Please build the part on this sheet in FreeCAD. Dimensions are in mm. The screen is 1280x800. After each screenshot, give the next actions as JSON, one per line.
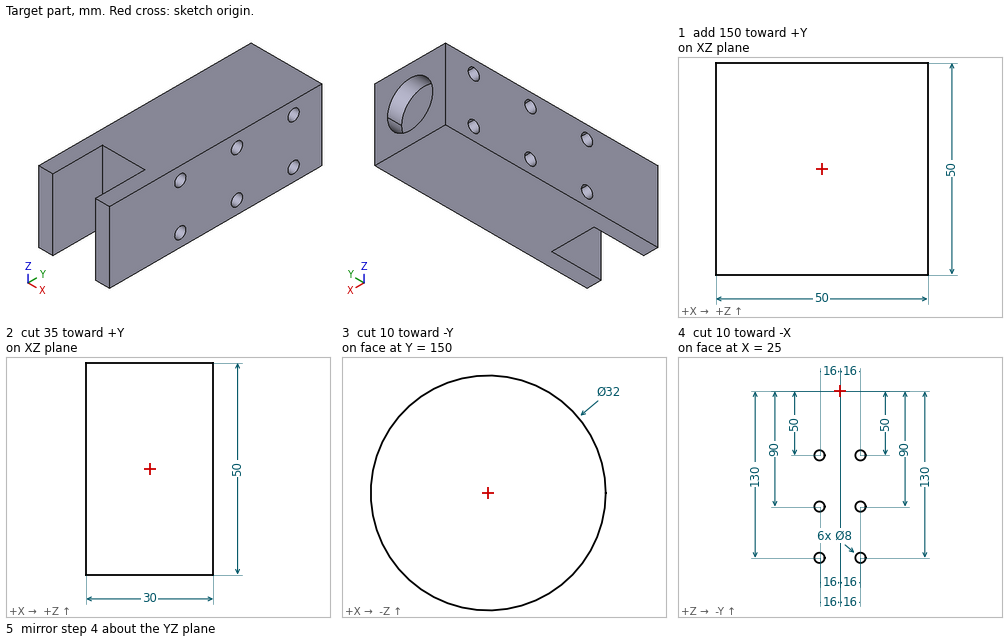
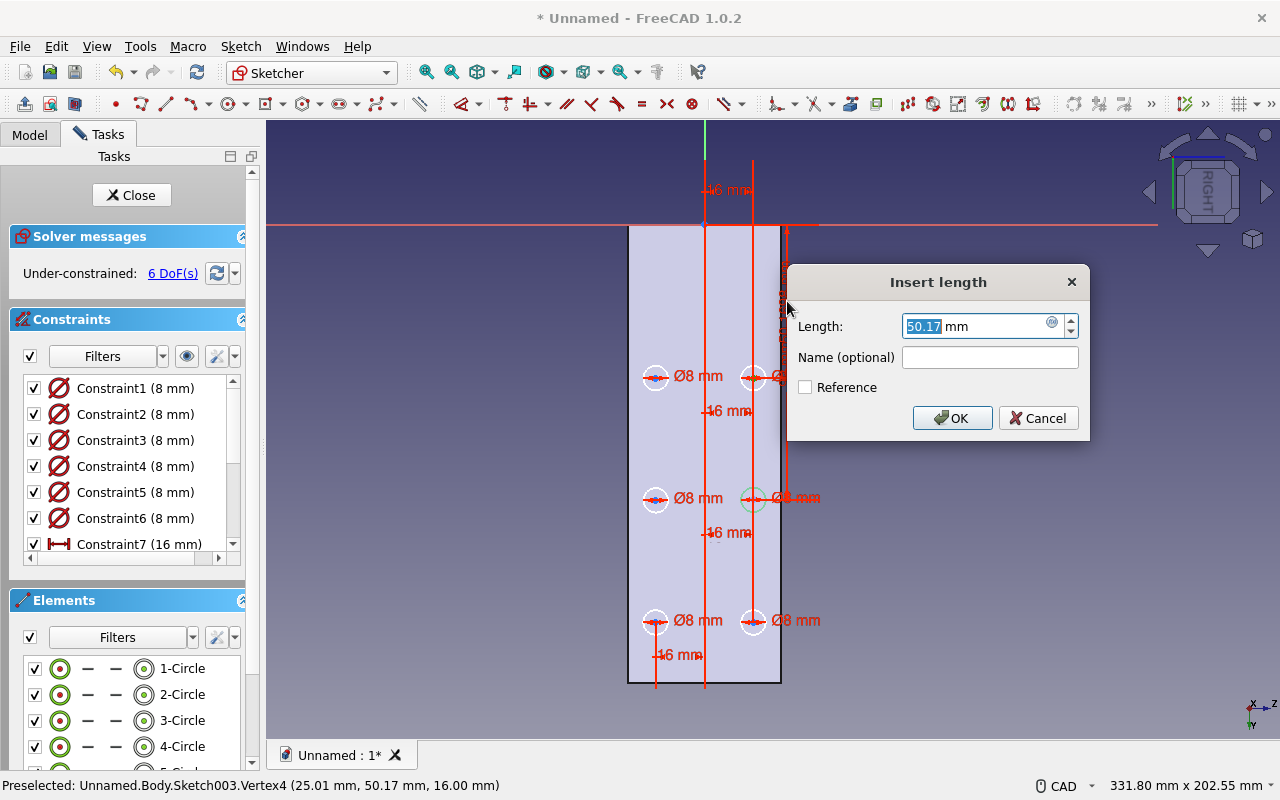
{"action": "type", "text": "50"}
{"action": "key", "text": "Return"}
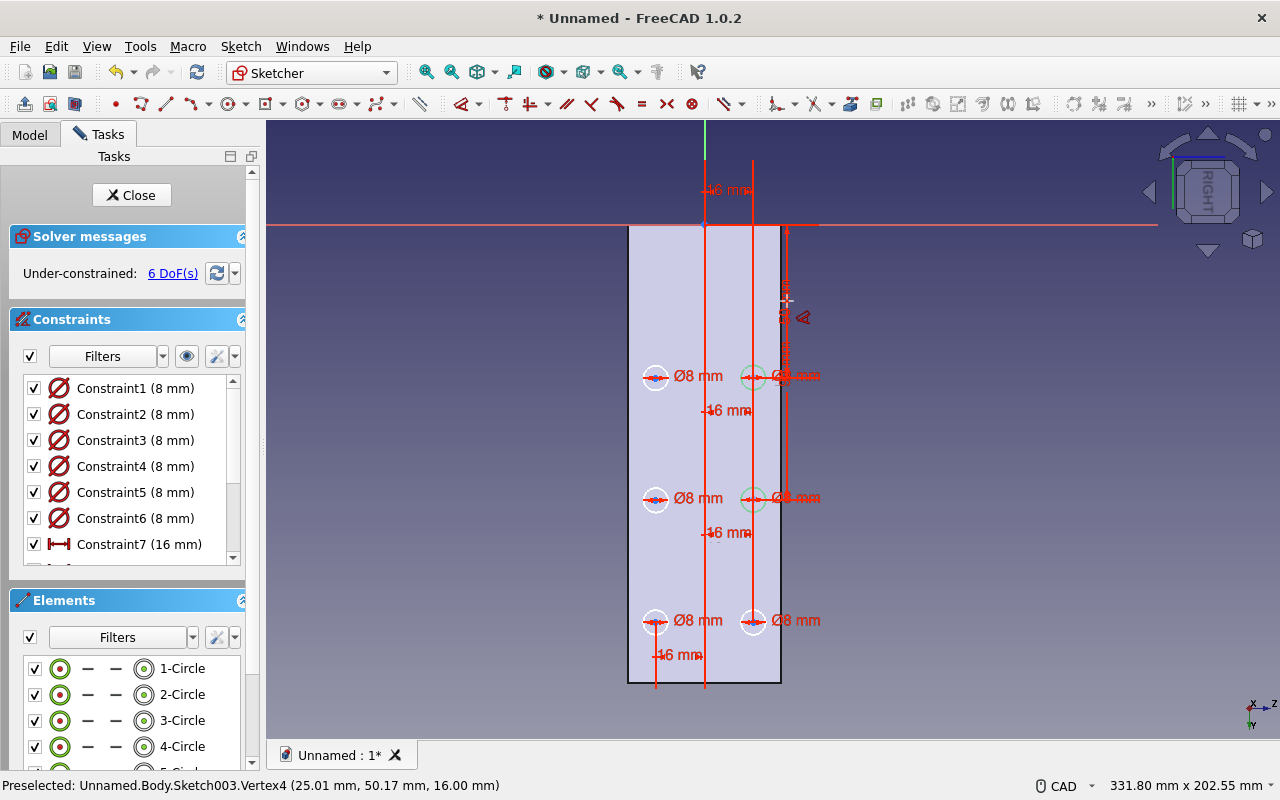
{"action": "left_click", "coordinate": [656, 378]}
{"action": "left_click", "coordinate": [680, 167]}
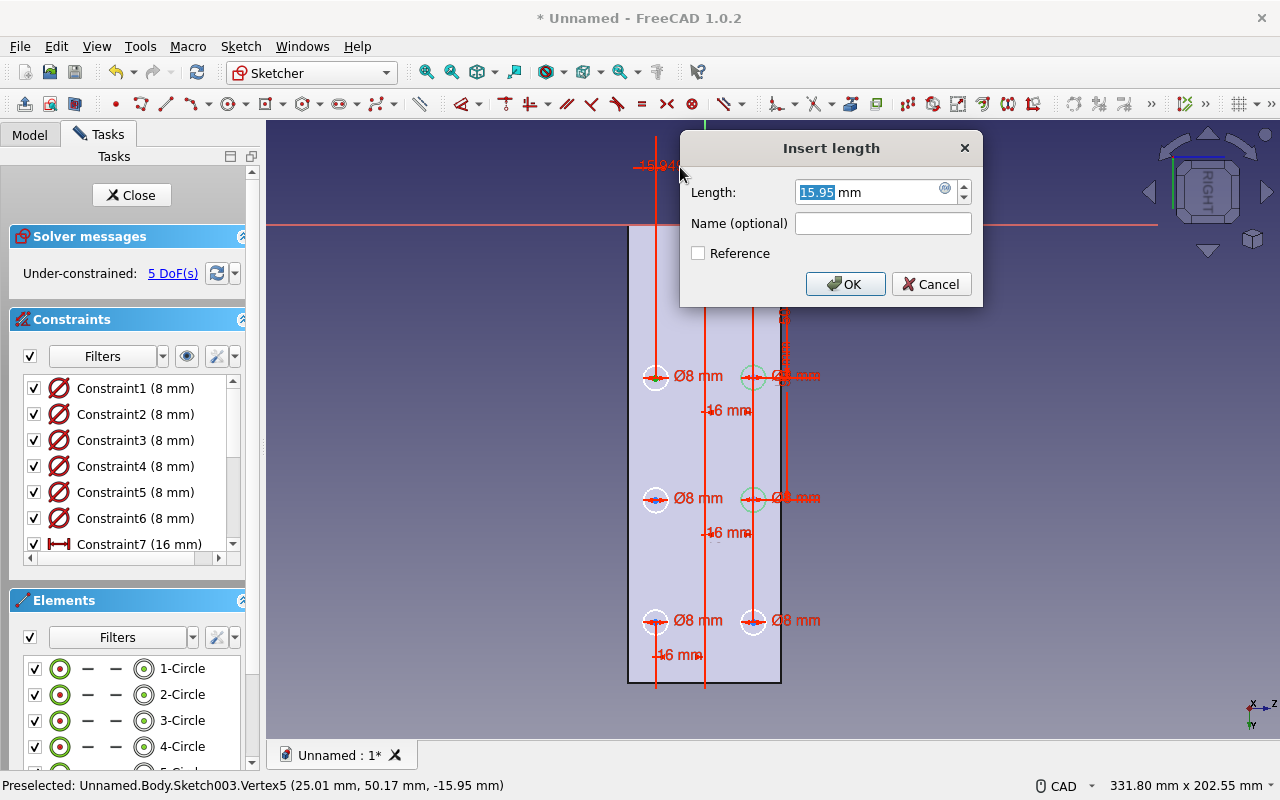
{"action": "type", "text": "16"}
{"action": "key", "text": "Return"}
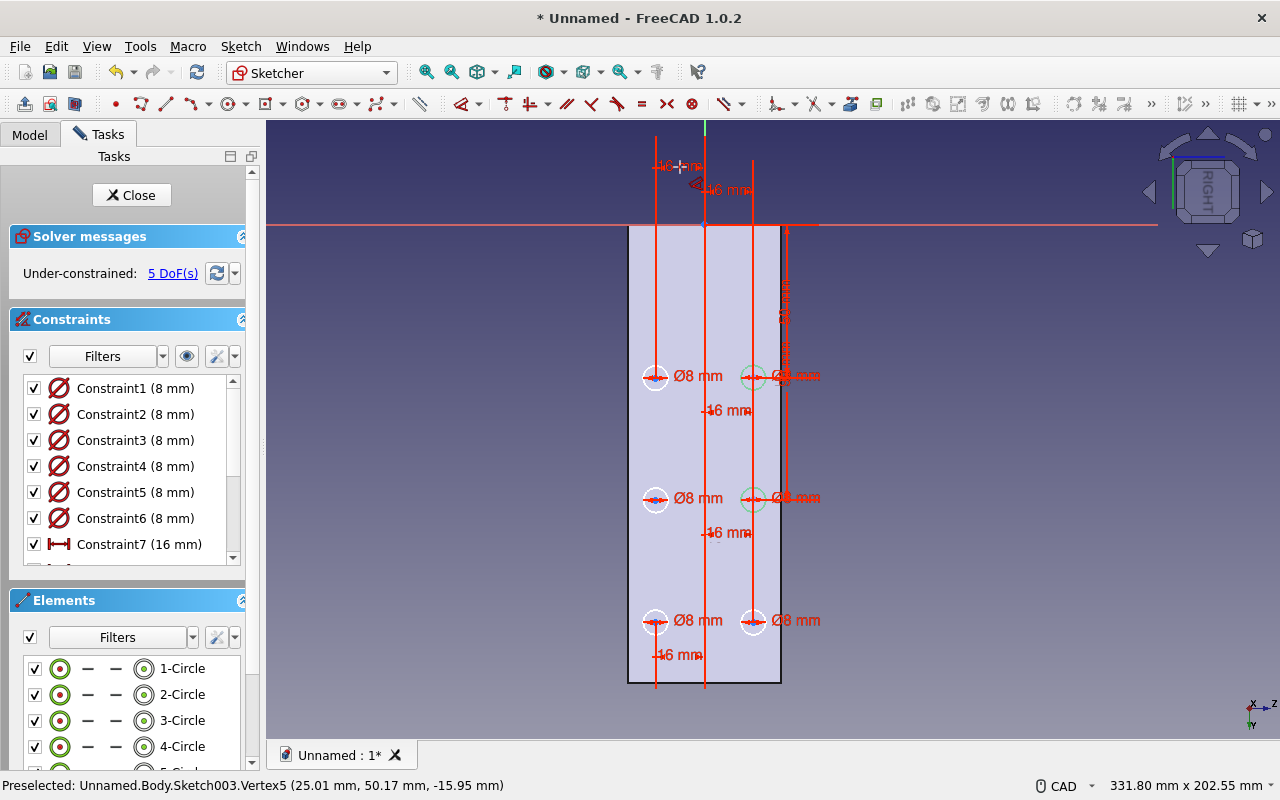
{"action": "left_click", "coordinate": [656, 378]}
{"action": "left_click", "coordinate": [622, 301]}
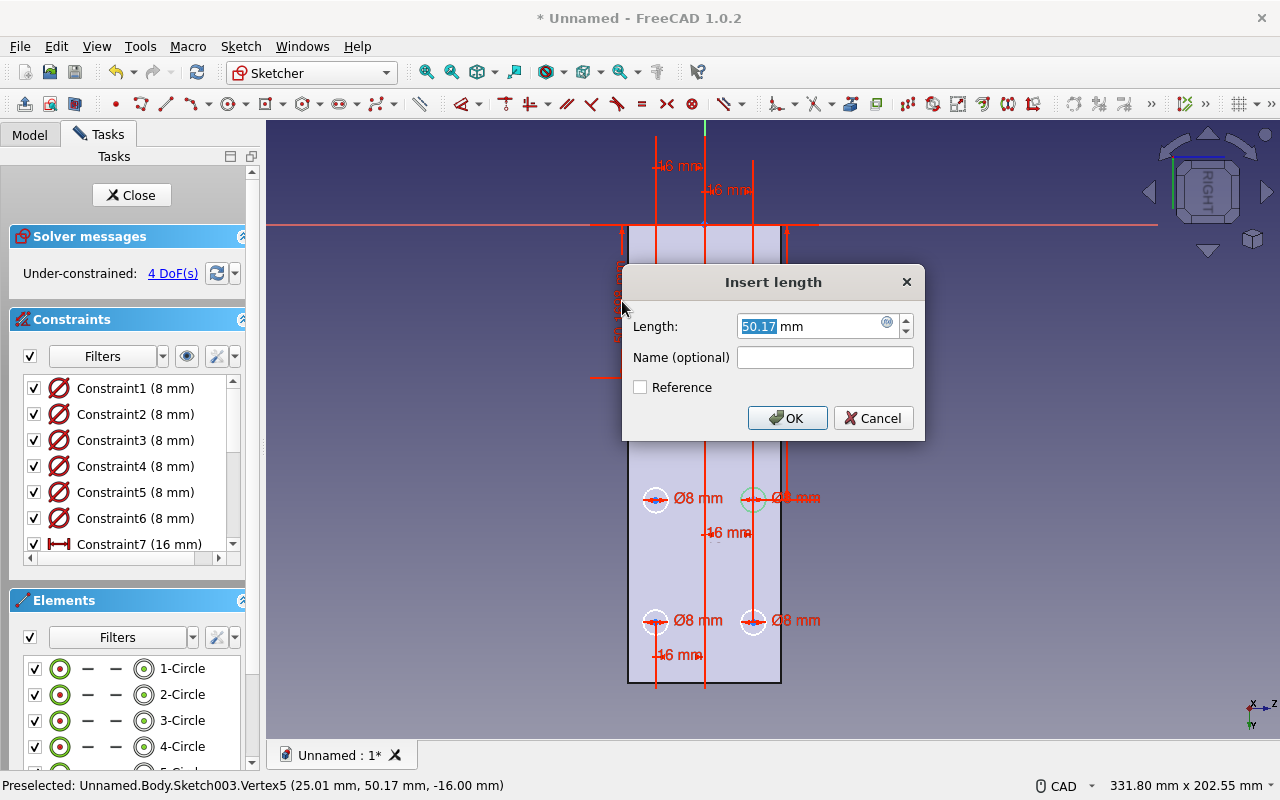
{"action": "type", "text": "50"}
{"action": "key", "text": "Return"}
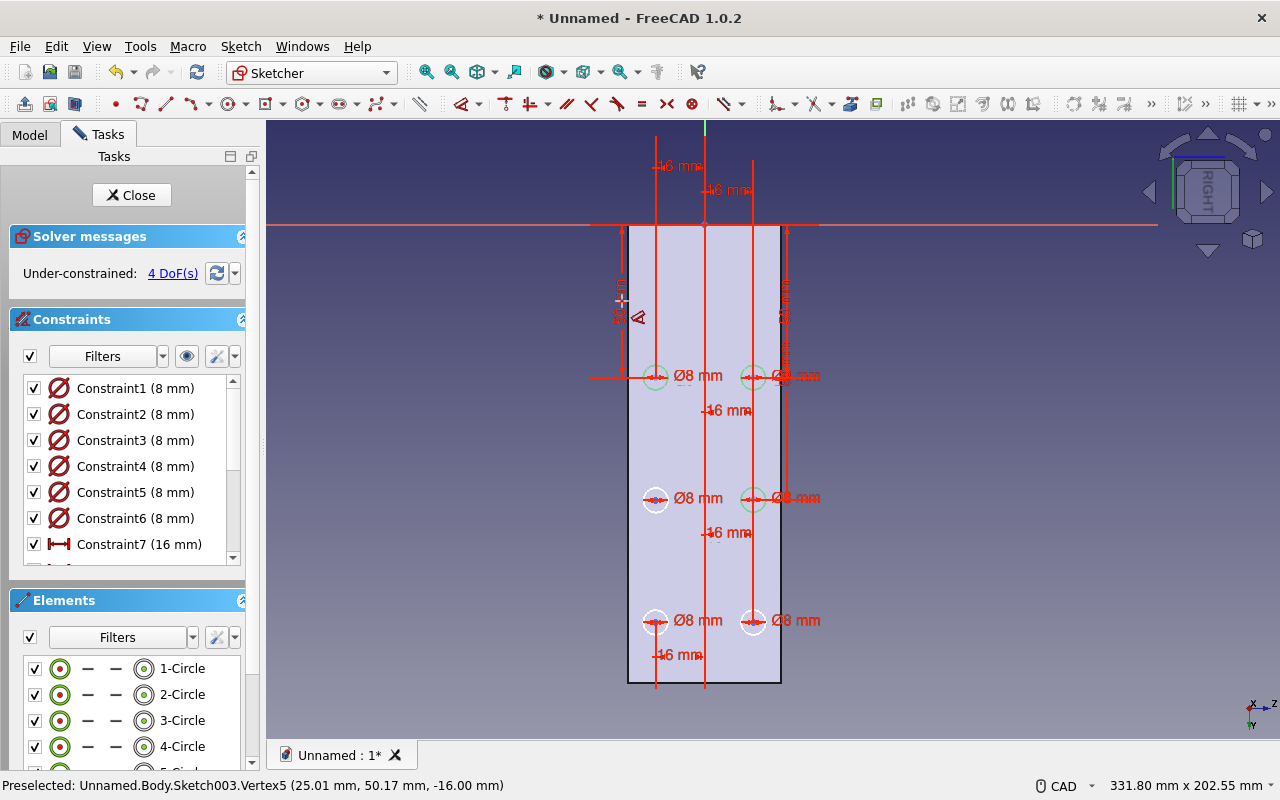
{"action": "left_click", "coordinate": [656, 500]}
{"action": "left_click", "coordinate": [680, 558]}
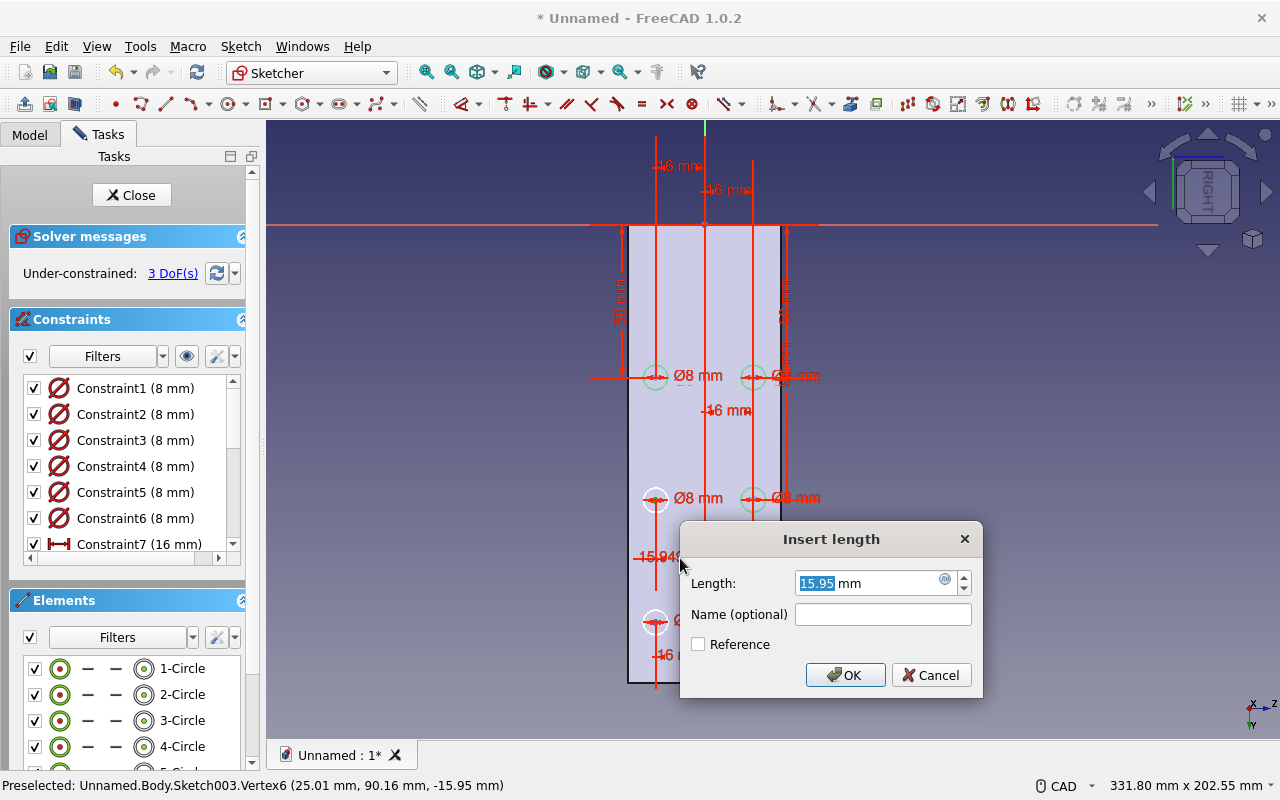
{"action": "type", "text": "16"}
{"action": "key", "text": "Return"}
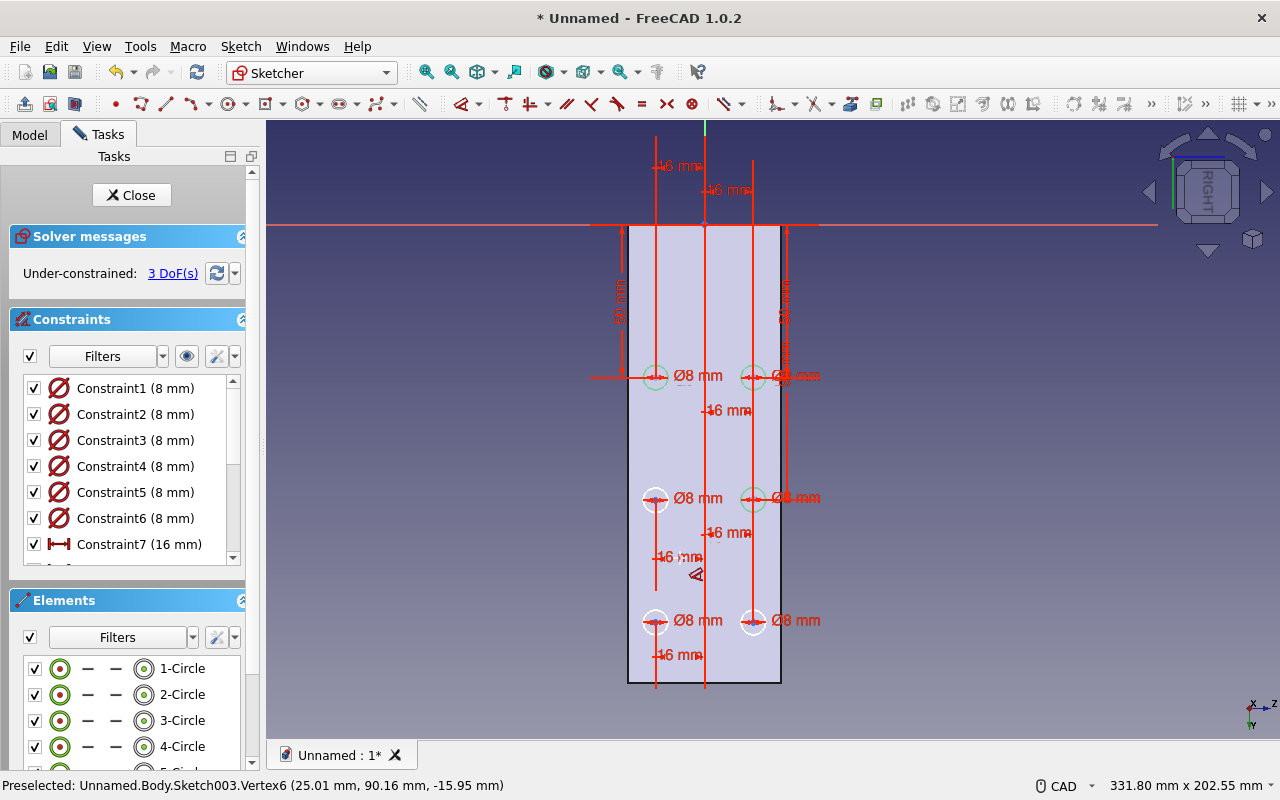
{"action": "left_click", "coordinate": [656, 500]}
{"action": "left_click", "coordinate": [622, 363]}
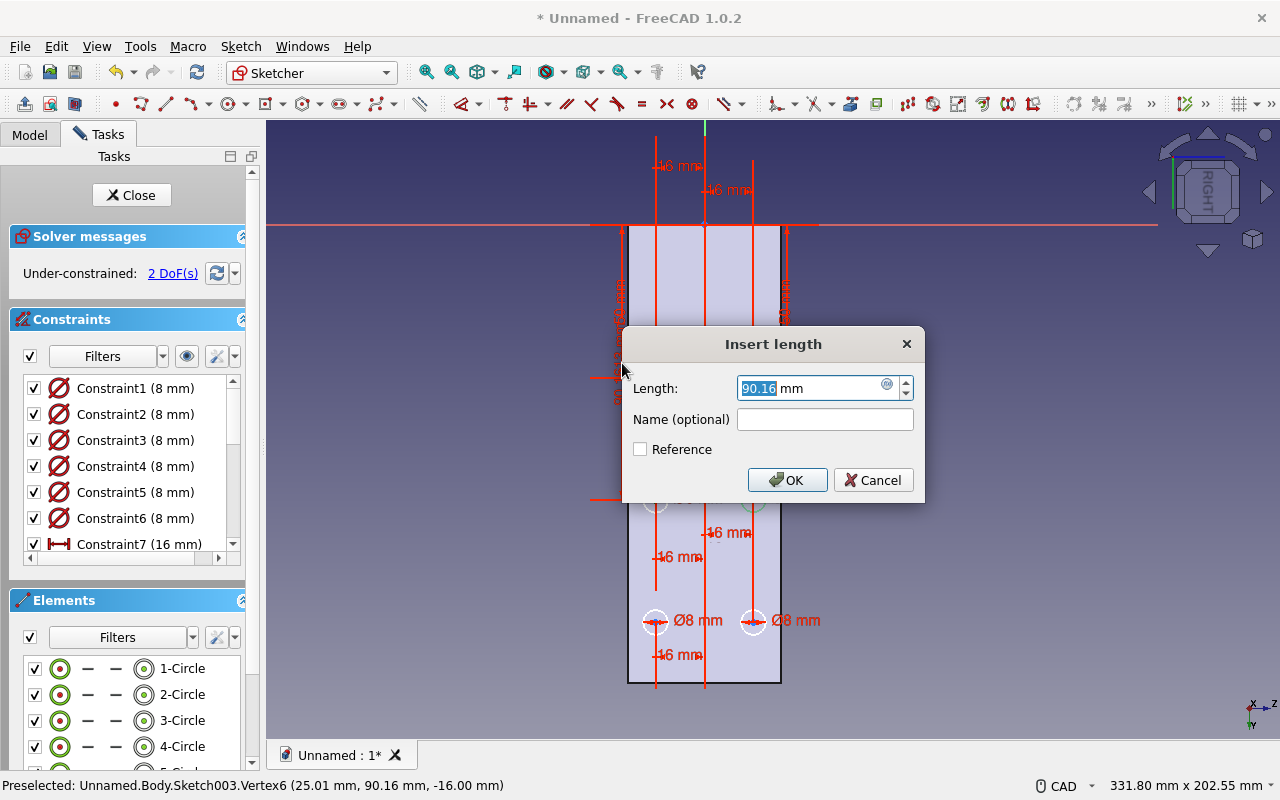
{"action": "type", "text": "90"}
{"action": "key", "text": "Return"}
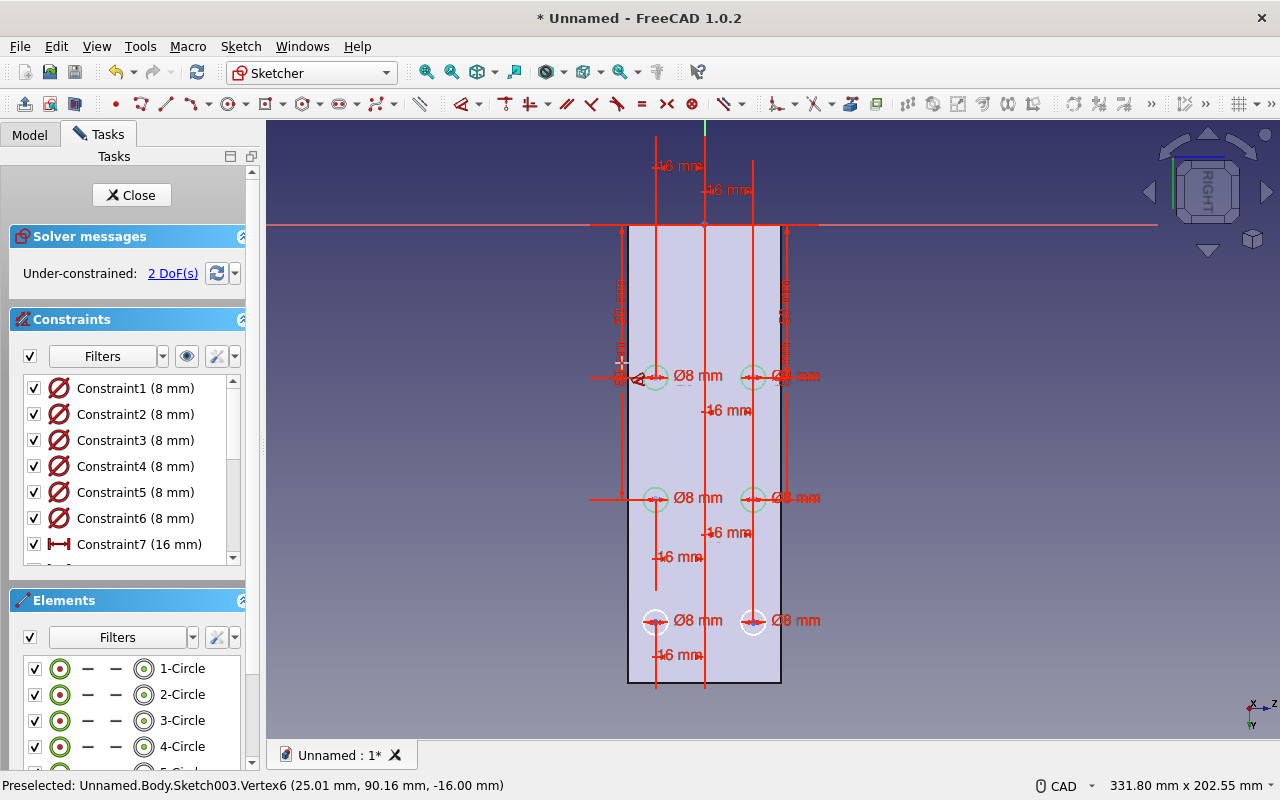
{"action": "left_click", "coordinate": [753, 622]}
{"action": "left_click", "coordinate": [787, 332]}